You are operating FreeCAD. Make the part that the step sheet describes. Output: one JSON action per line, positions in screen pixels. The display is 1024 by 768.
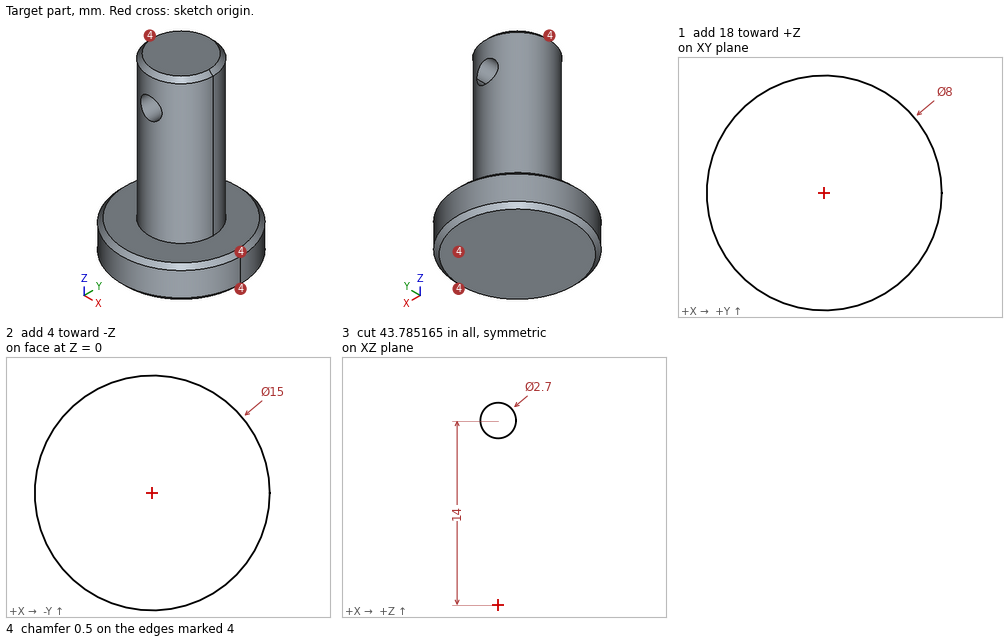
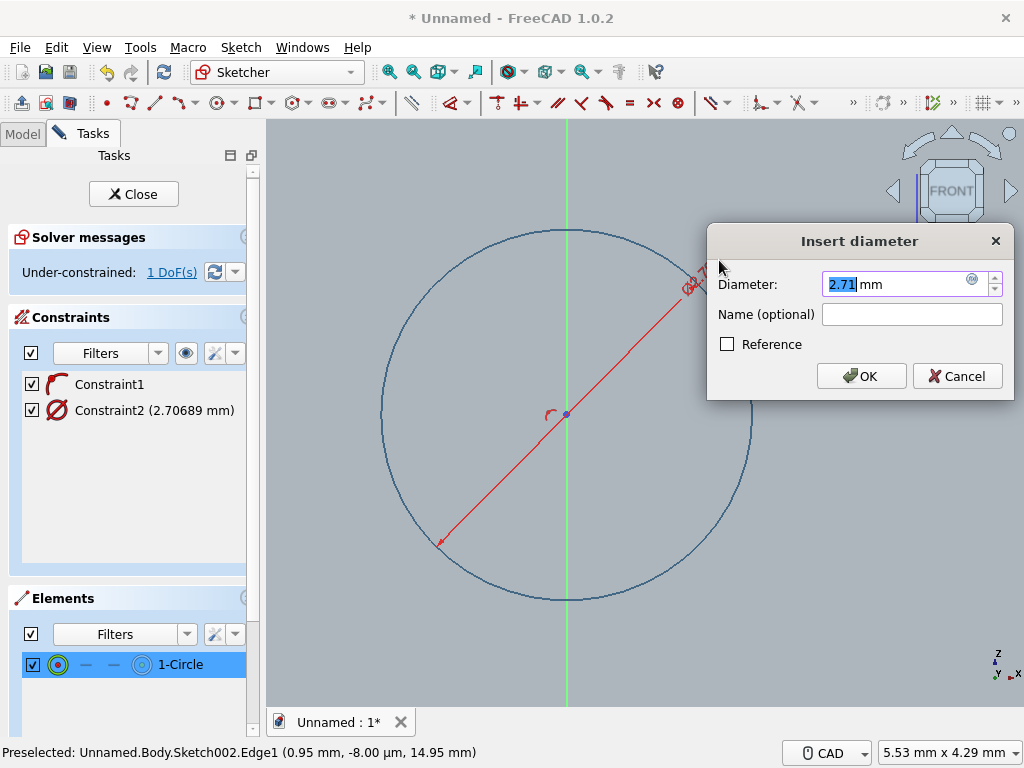
{"action": "type", "text": "2.7"}
{"action": "key", "text": "Return"}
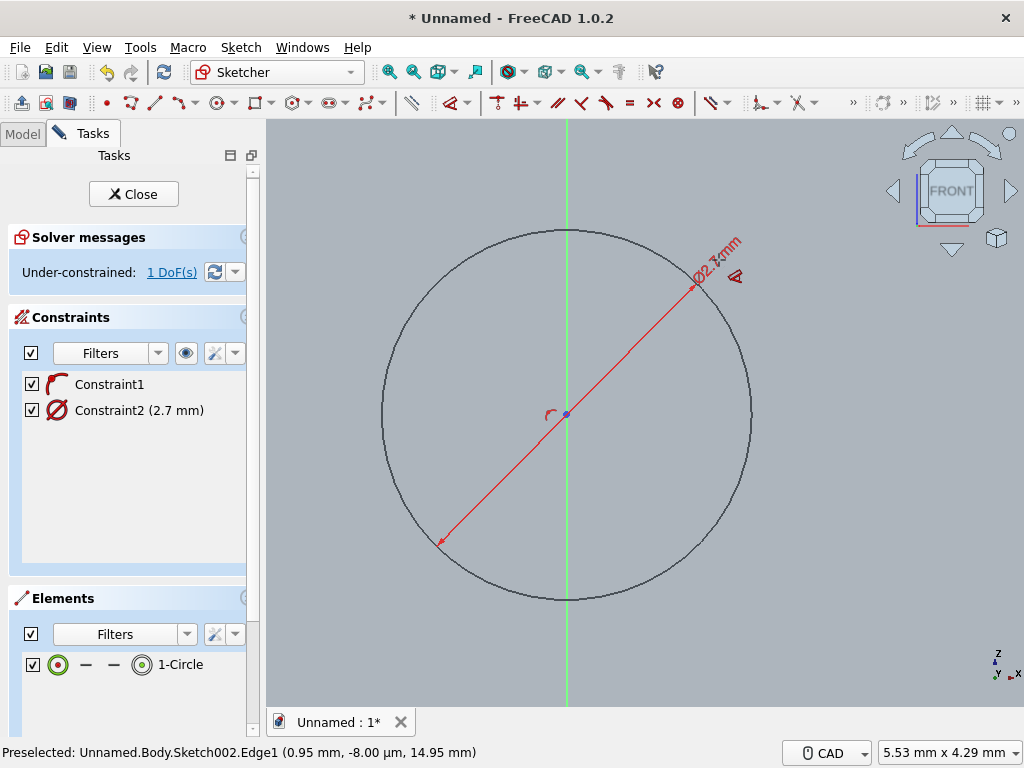
{"action": "left_click", "coordinate": [567, 415]}
{"action": "left_click", "coordinate": [601, 547]}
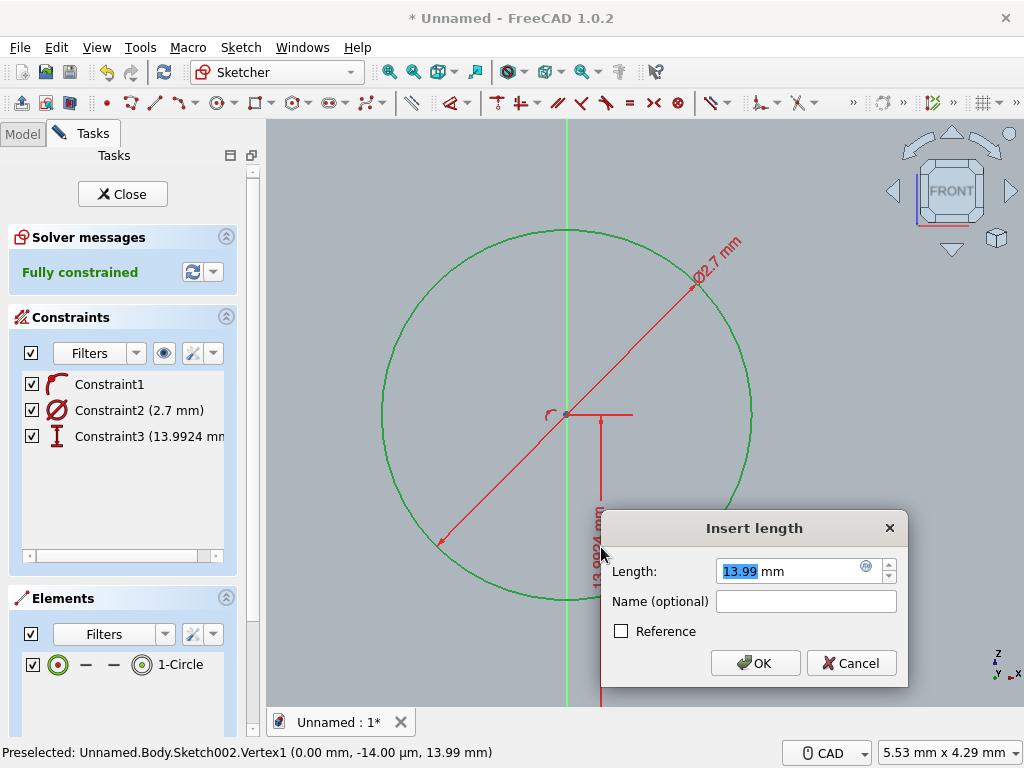
{"action": "type", "text": "14"}
{"action": "key", "text": "Return"}
{"action": "key", "text": "Escape"}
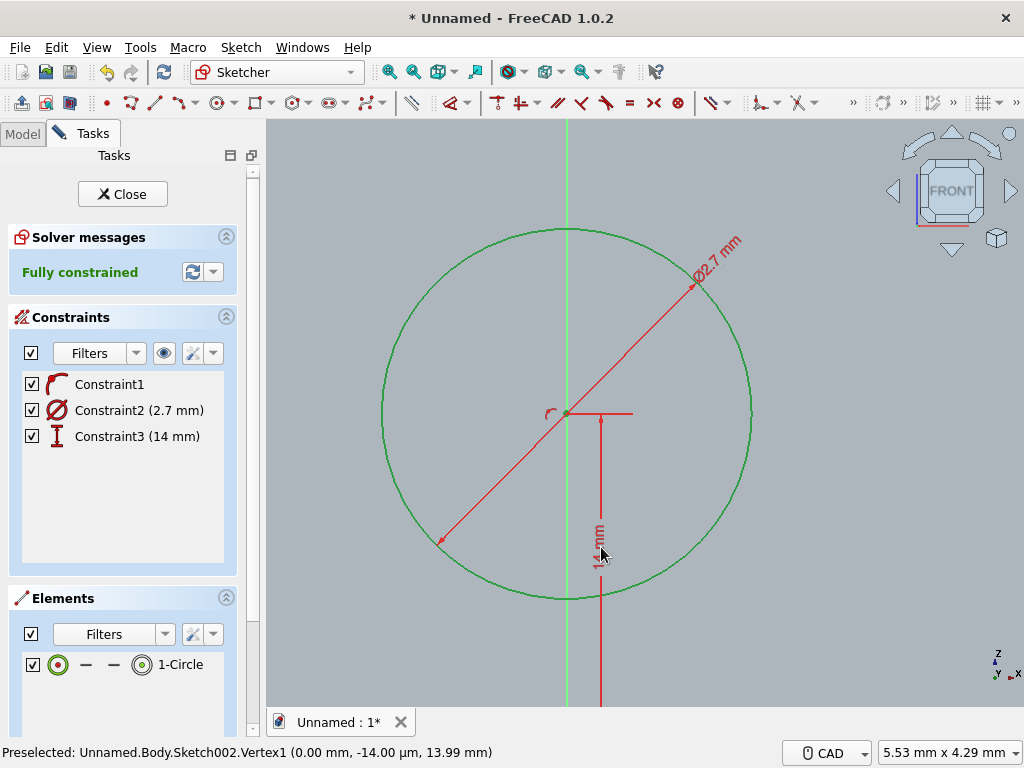
{"action": "left_click", "coordinate": [123, 194]}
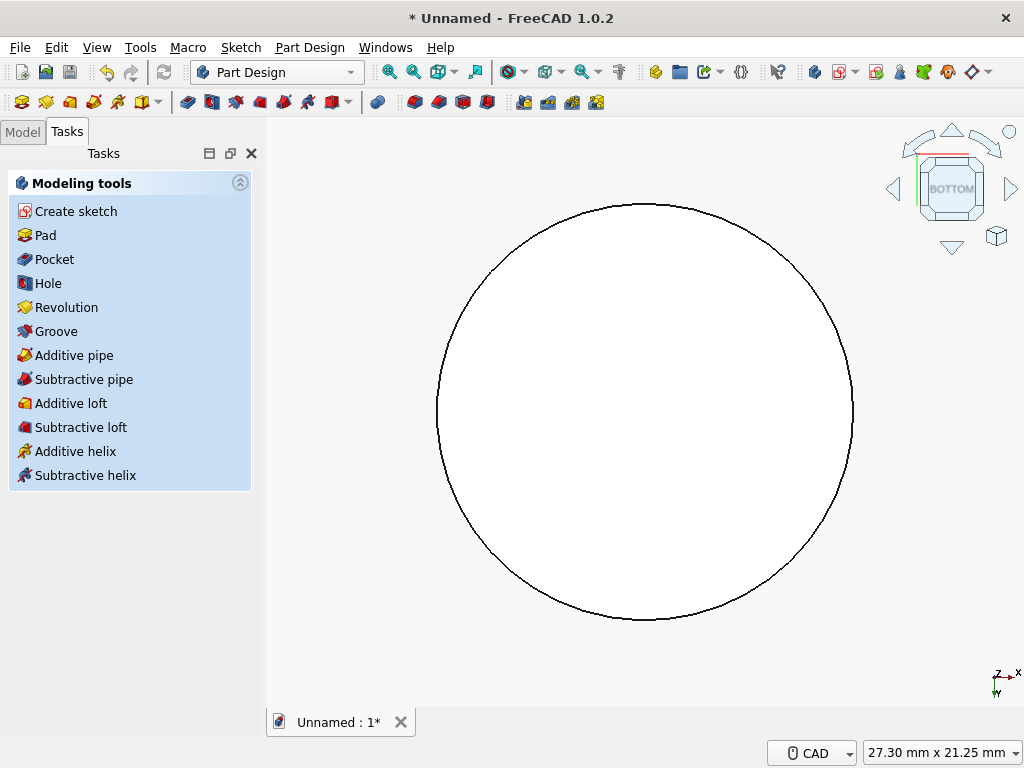
{"action": "left_click", "coordinate": [188, 102]}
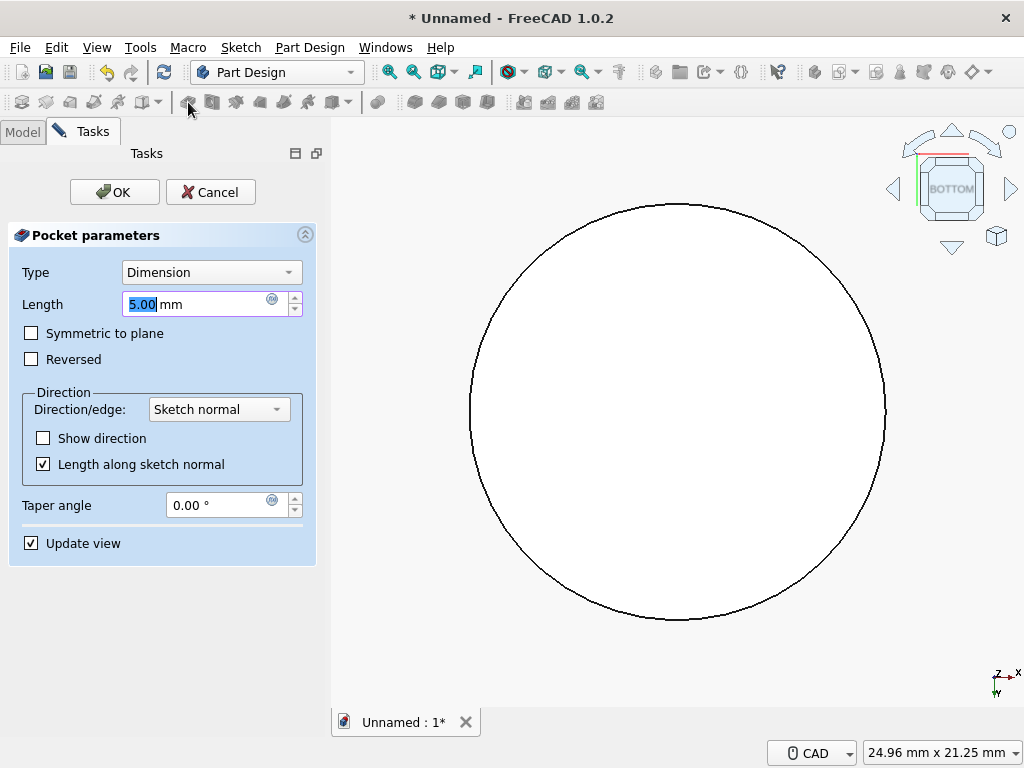
{"action": "type", "text": "43.785165"}
{"action": "key", "text": "Tab"}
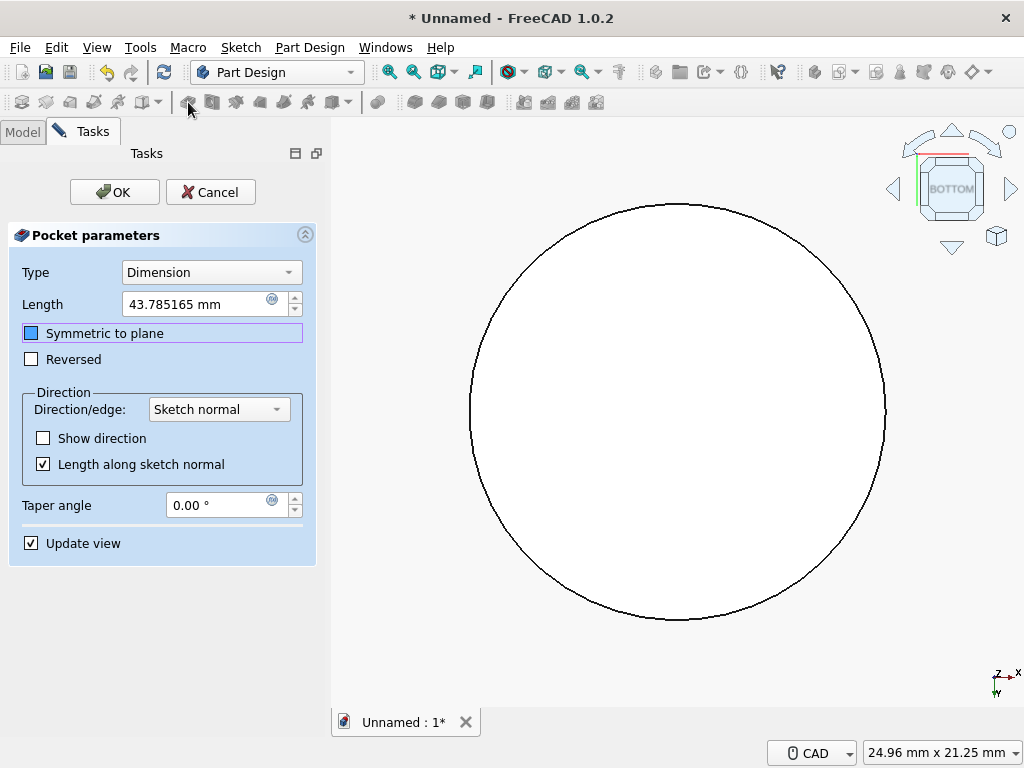
{"action": "left_click", "coordinate": [30, 333]}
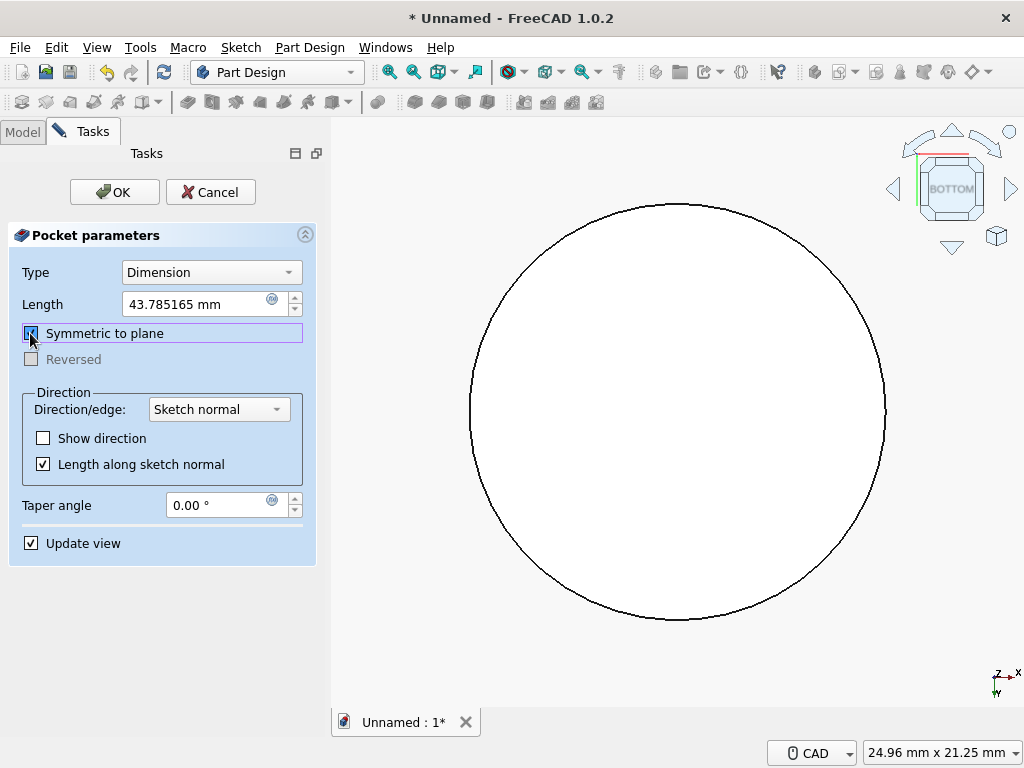
{"action": "left_click", "coordinate": [115, 192]}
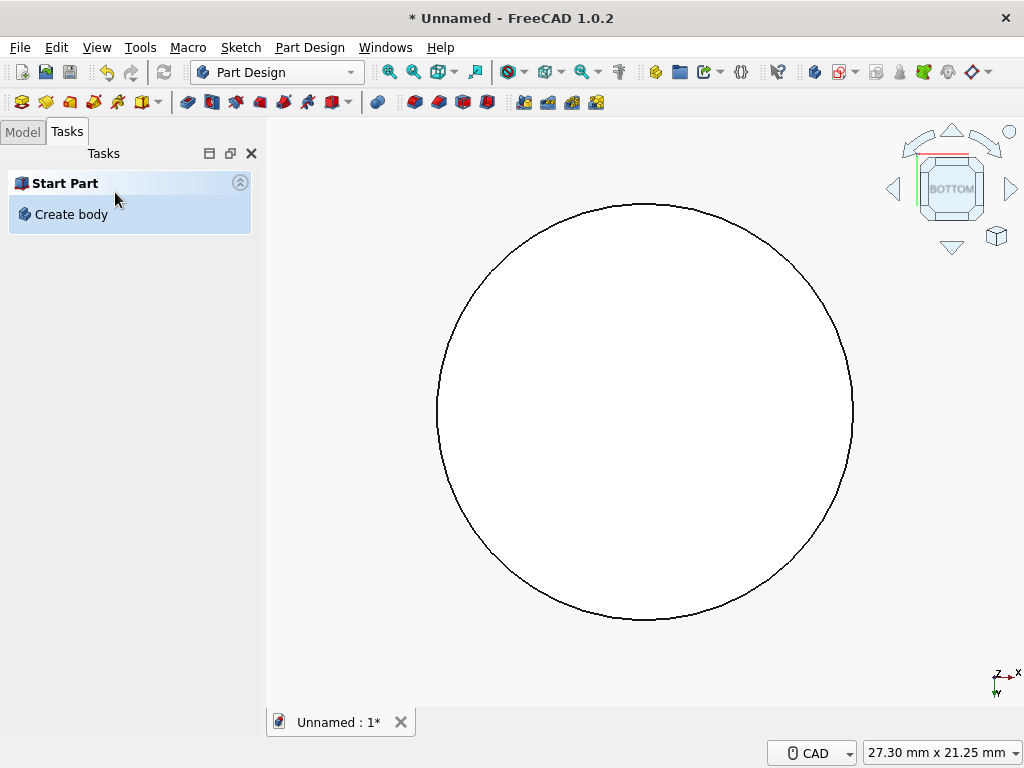
{"action": "left_click", "coordinate": [437, 411]}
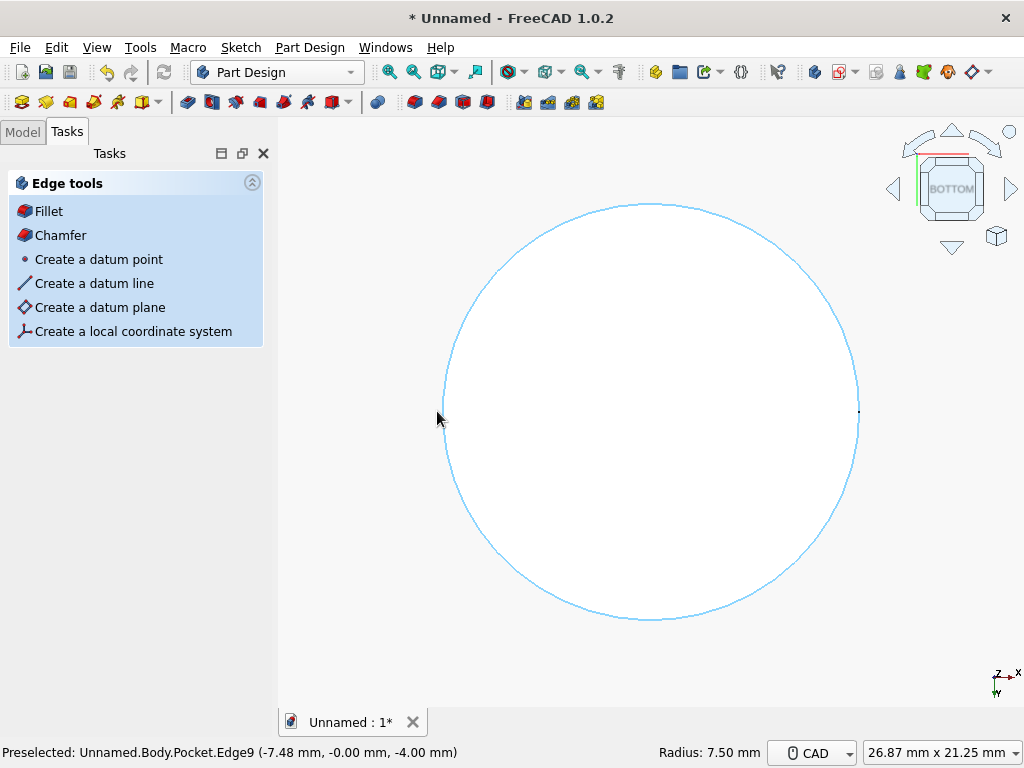
{"action": "key", "text": "0"}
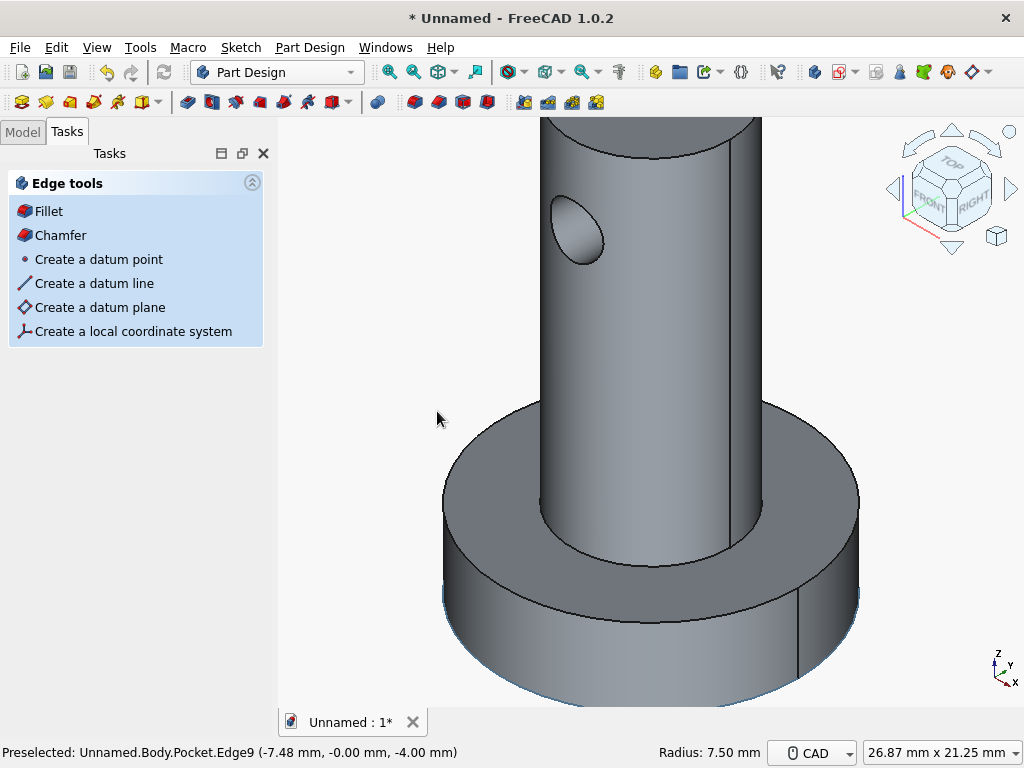
{"action": "left_click", "coordinate": [390, 72]}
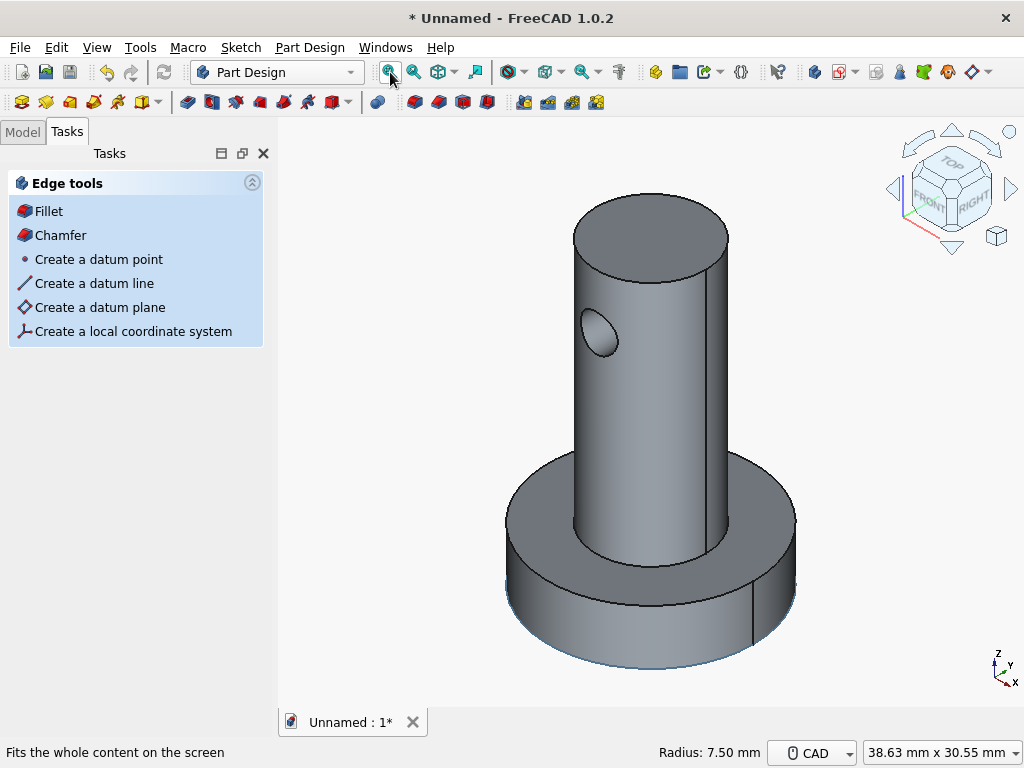
{"action": "left_click", "coordinate": [582, 258], "text": "ctrl"}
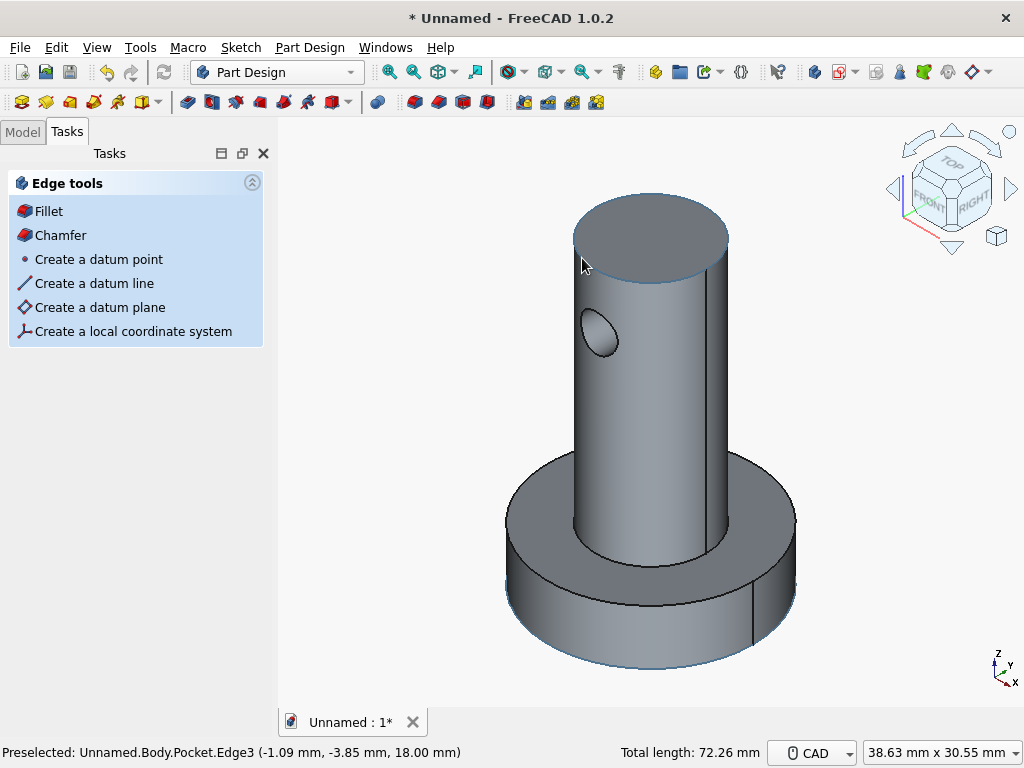
{"action": "left_click", "coordinate": [522, 559], "text": "ctrl"}